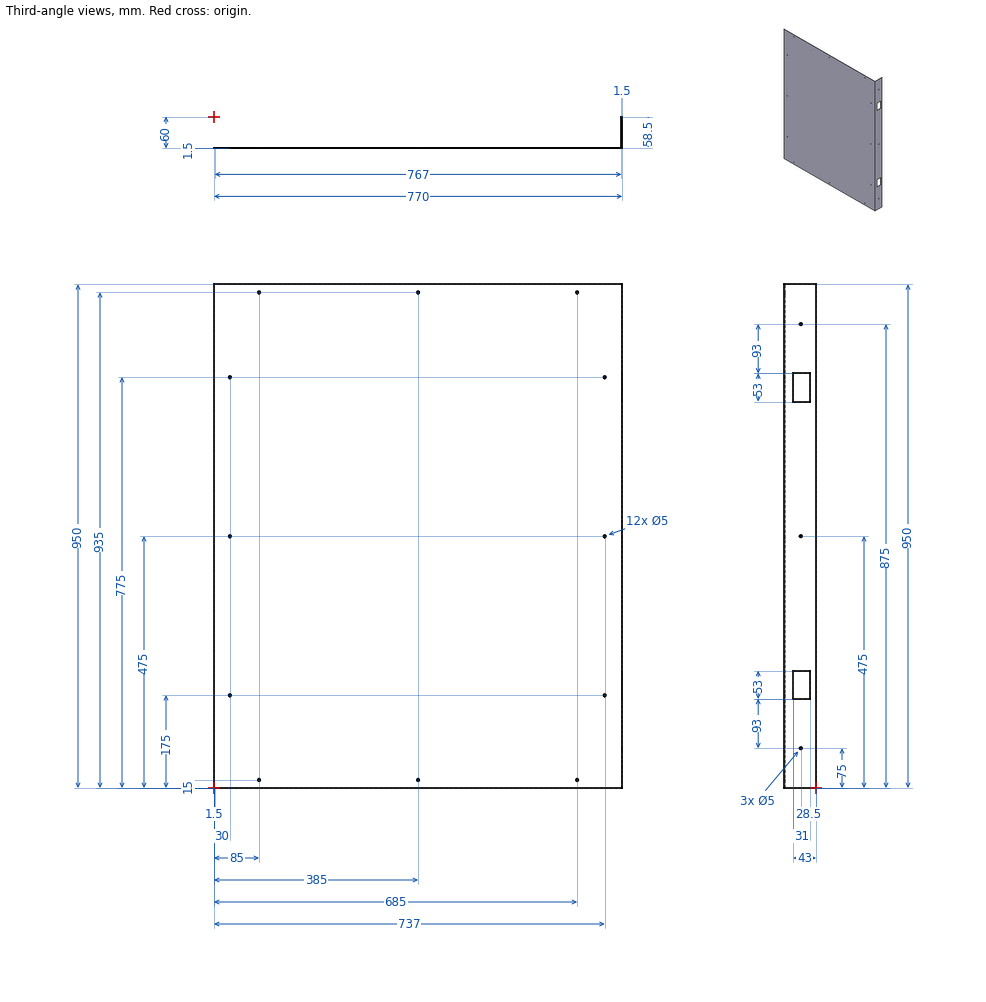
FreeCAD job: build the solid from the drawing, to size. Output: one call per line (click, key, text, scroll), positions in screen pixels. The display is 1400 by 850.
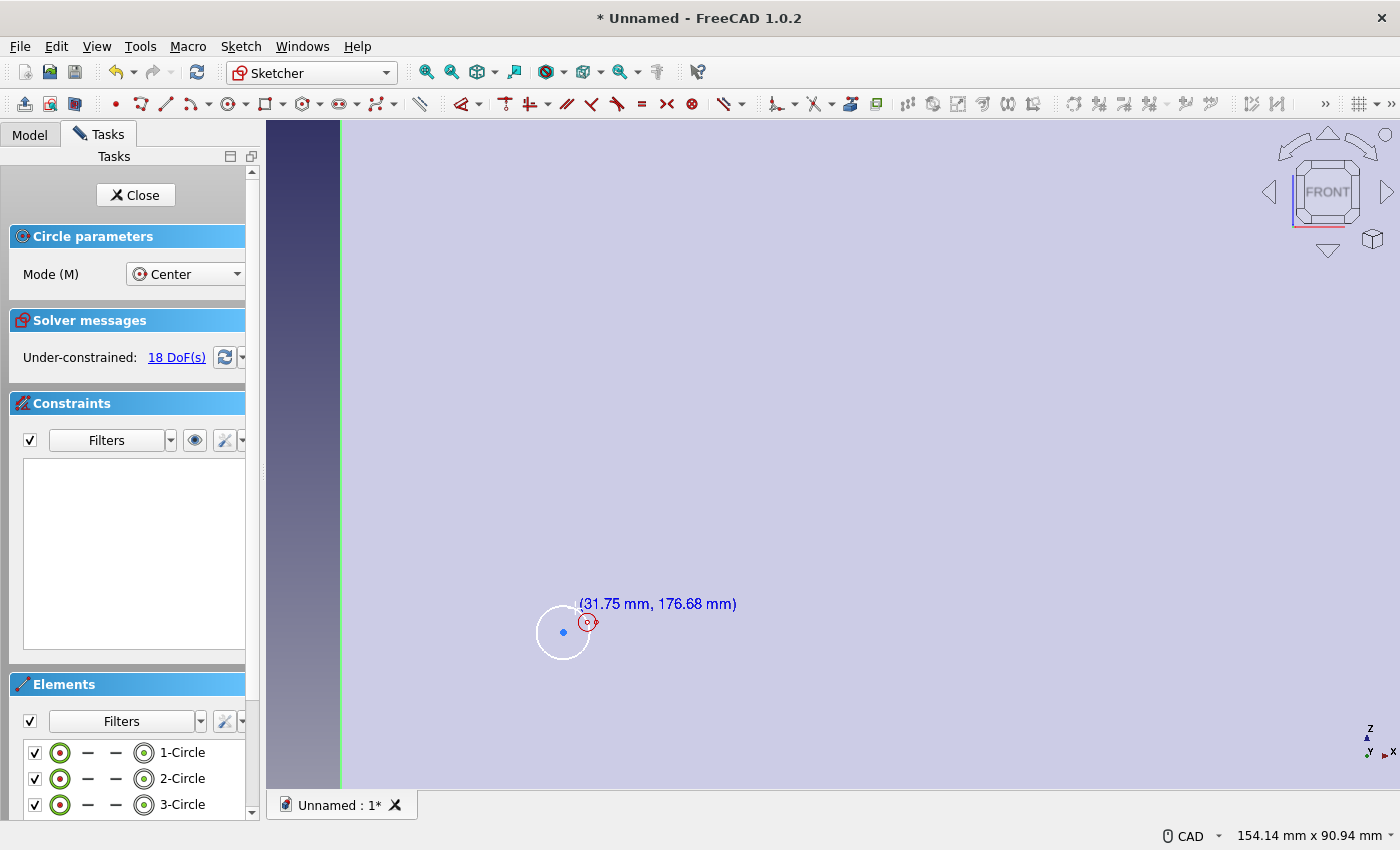
scroll(616, 584, down, 14)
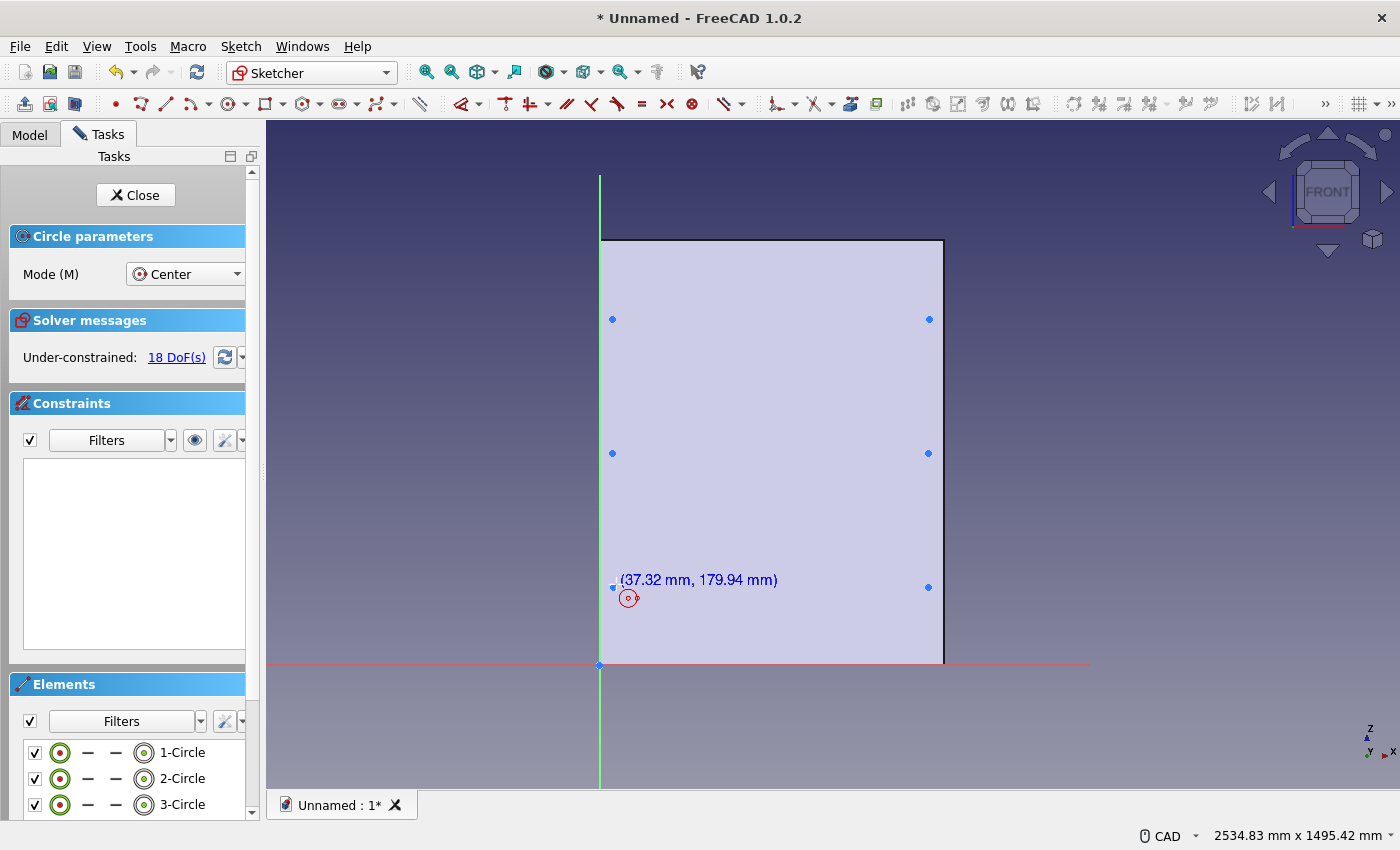
scroll(772, 247, up, 16)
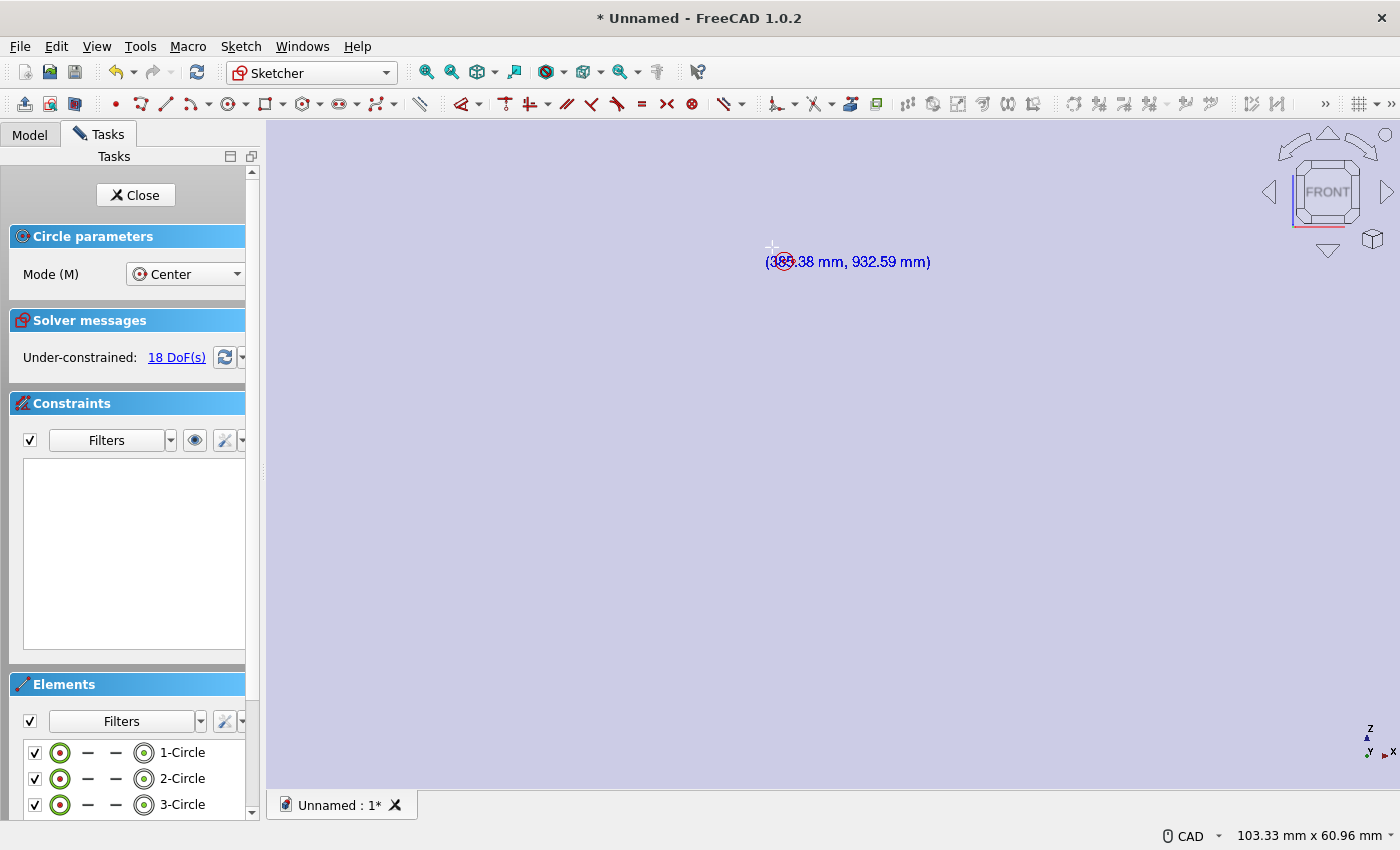
scroll(774, 198, down, 15)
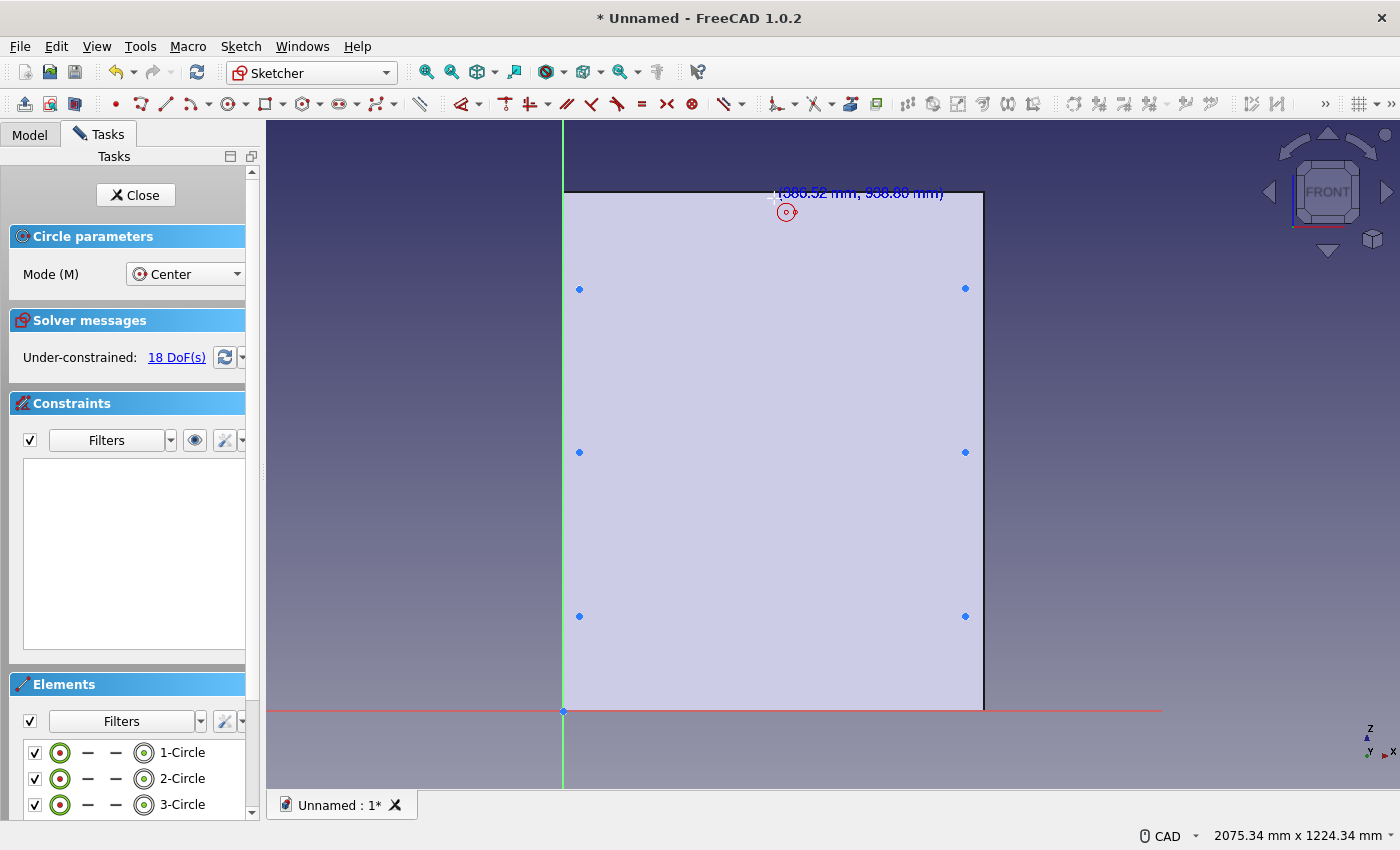
click(774, 200)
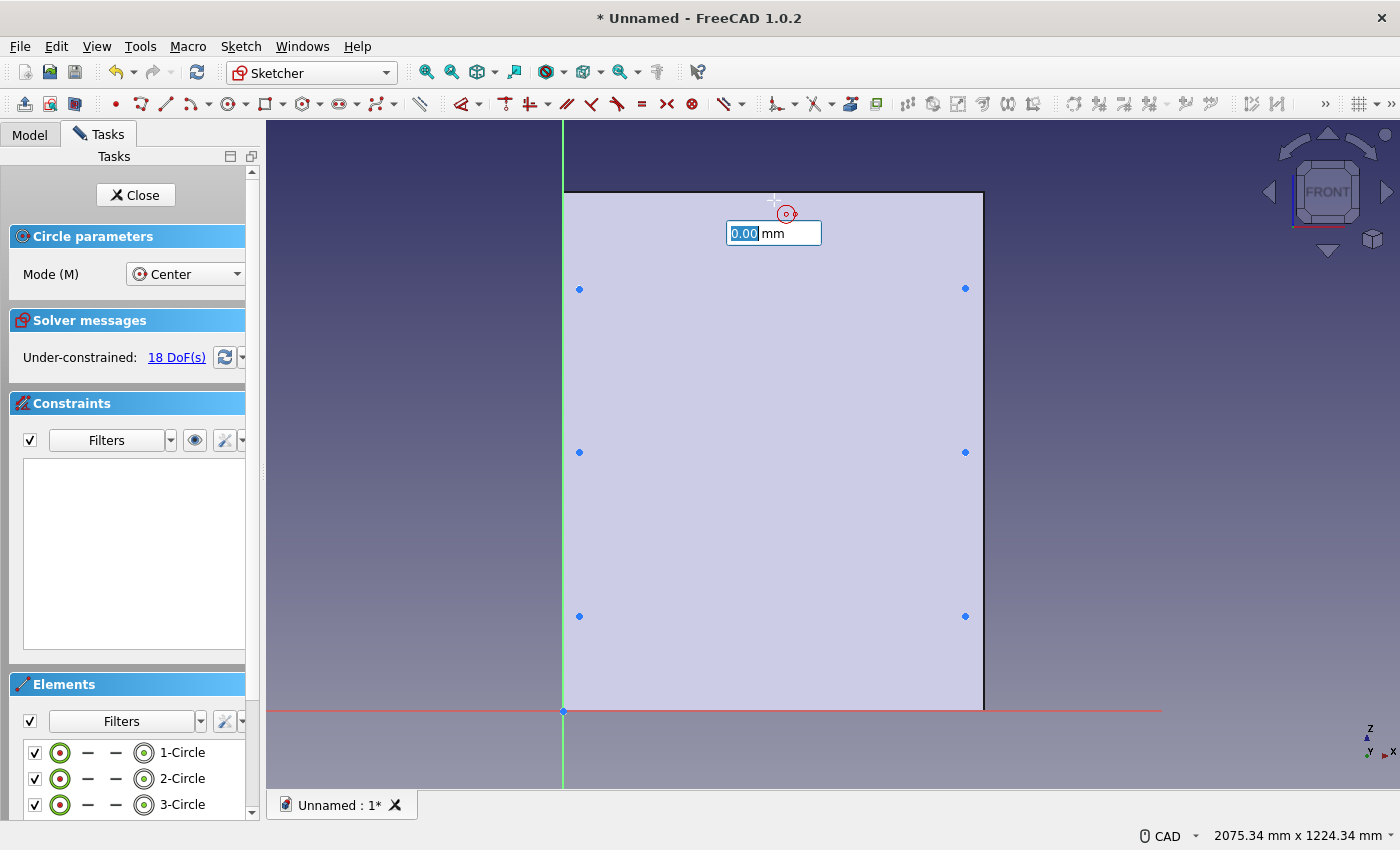
scroll(775, 199, up, 13)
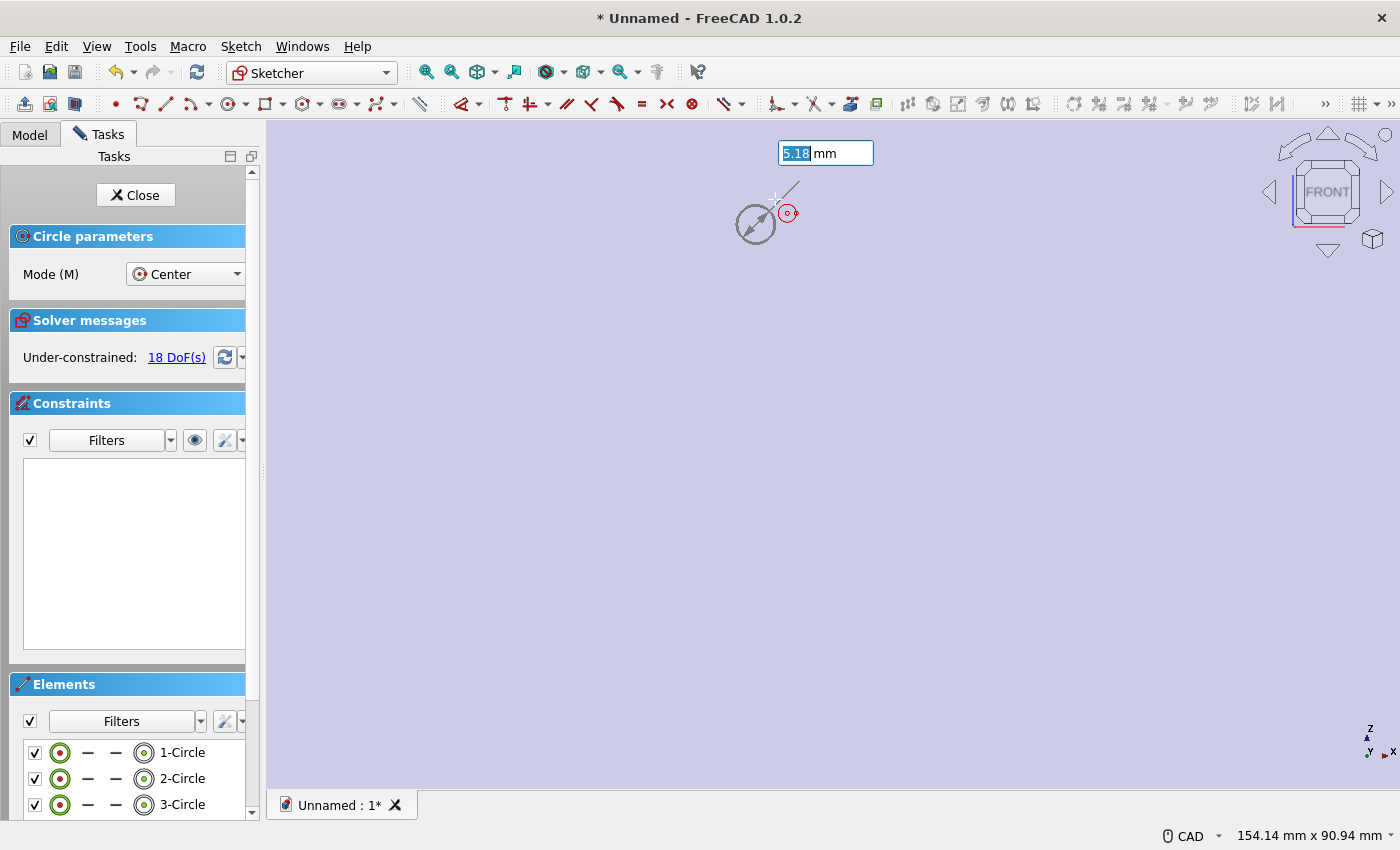
click(763, 201)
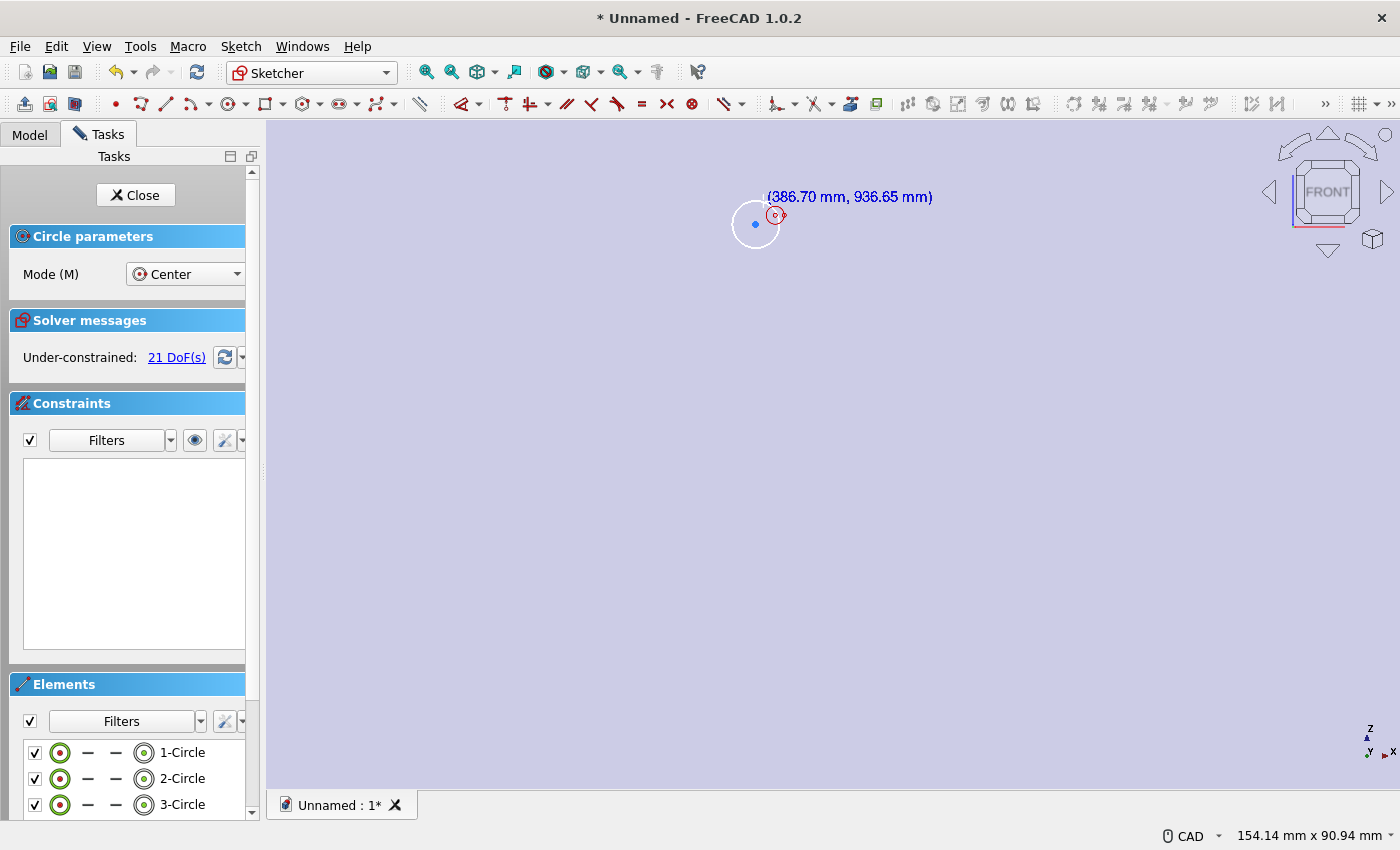
scroll(773, 248, down, 14)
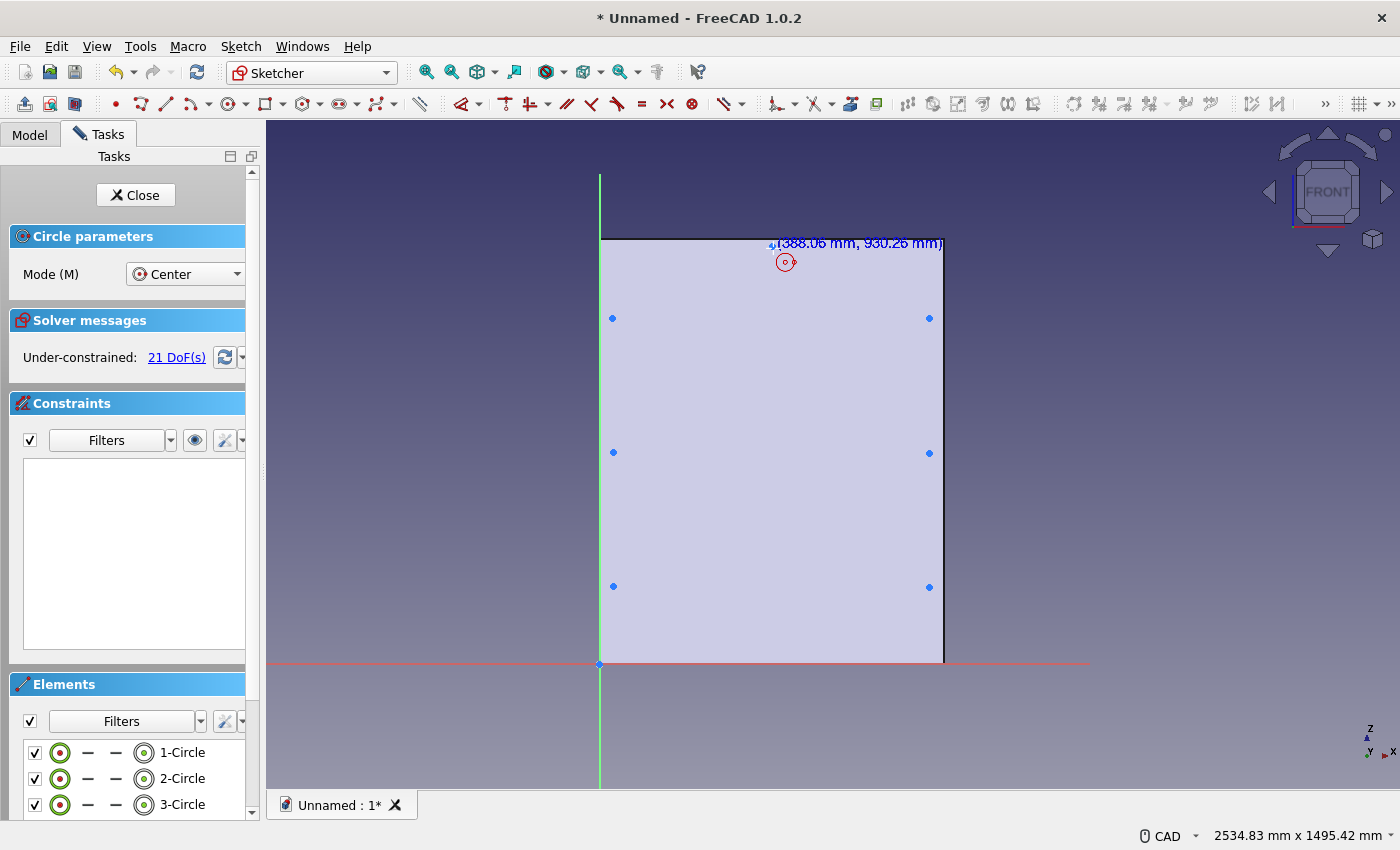
scroll(906, 246, up, 16)